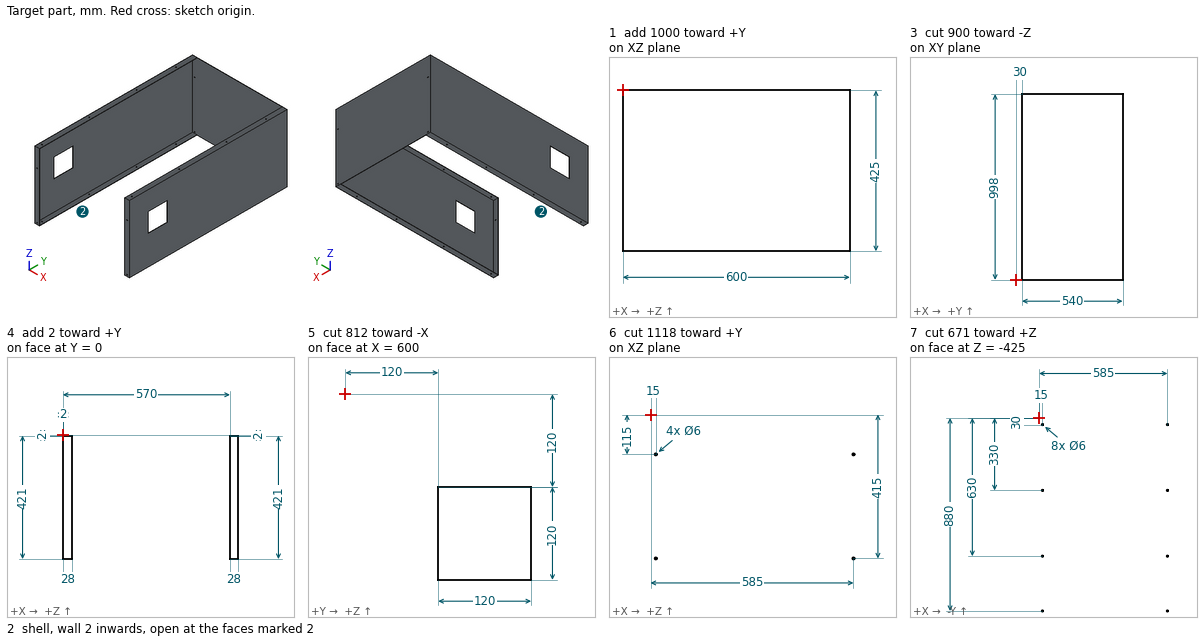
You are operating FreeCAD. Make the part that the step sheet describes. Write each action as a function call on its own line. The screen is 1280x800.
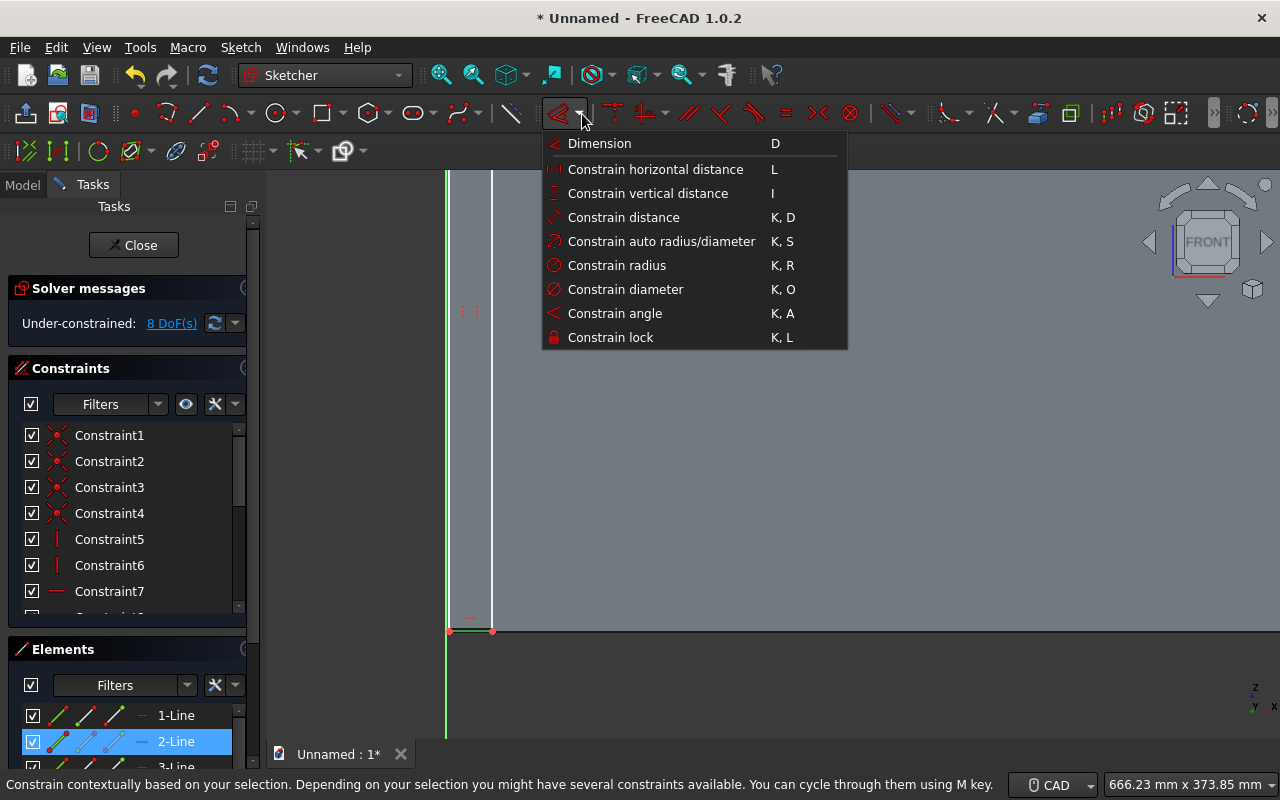
click(695, 169)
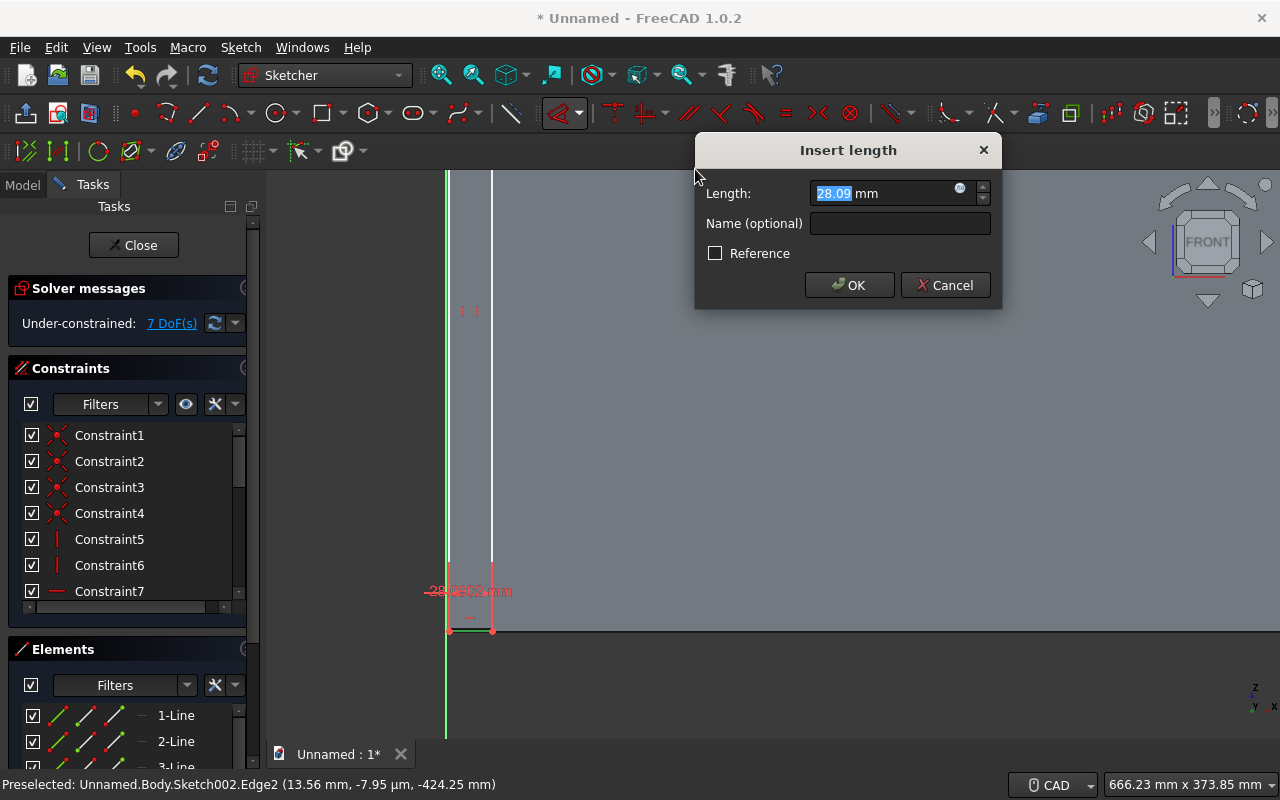
text(28)
key(Return)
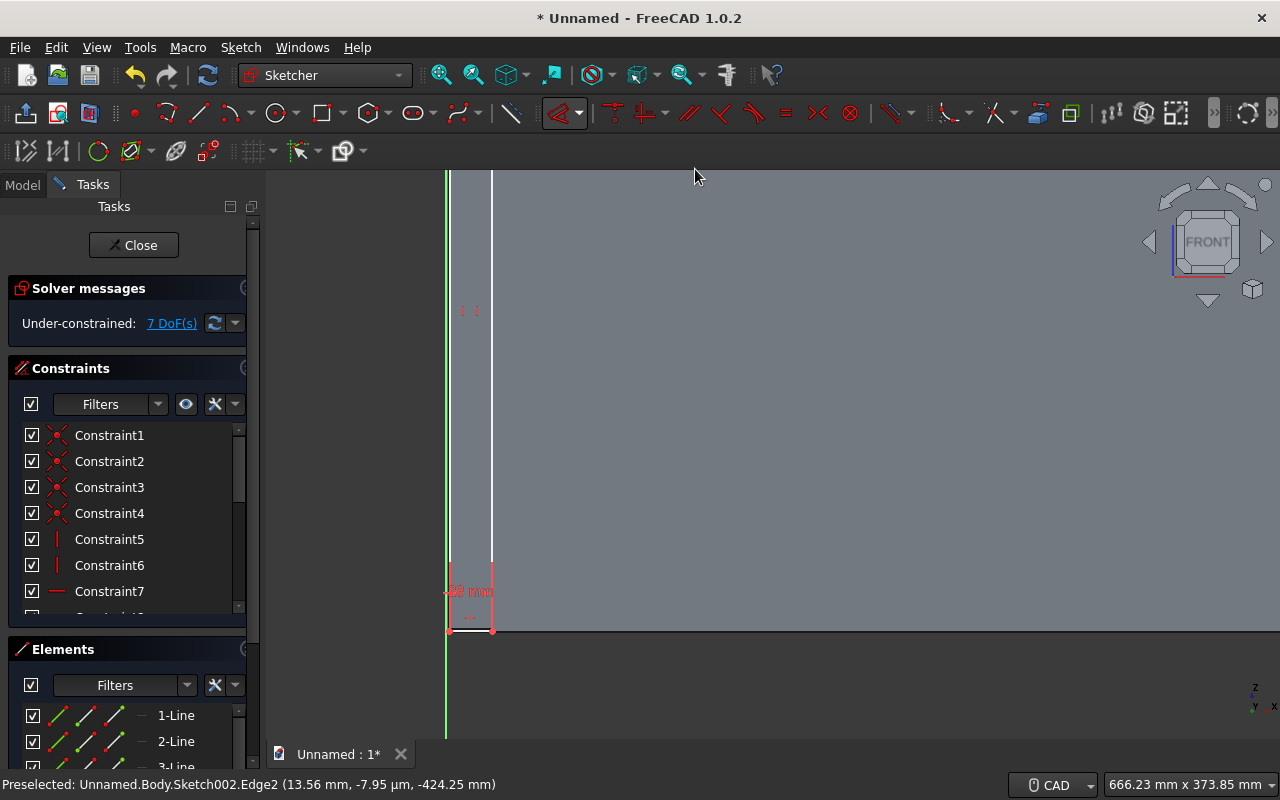
scroll(465, 633, down, 3)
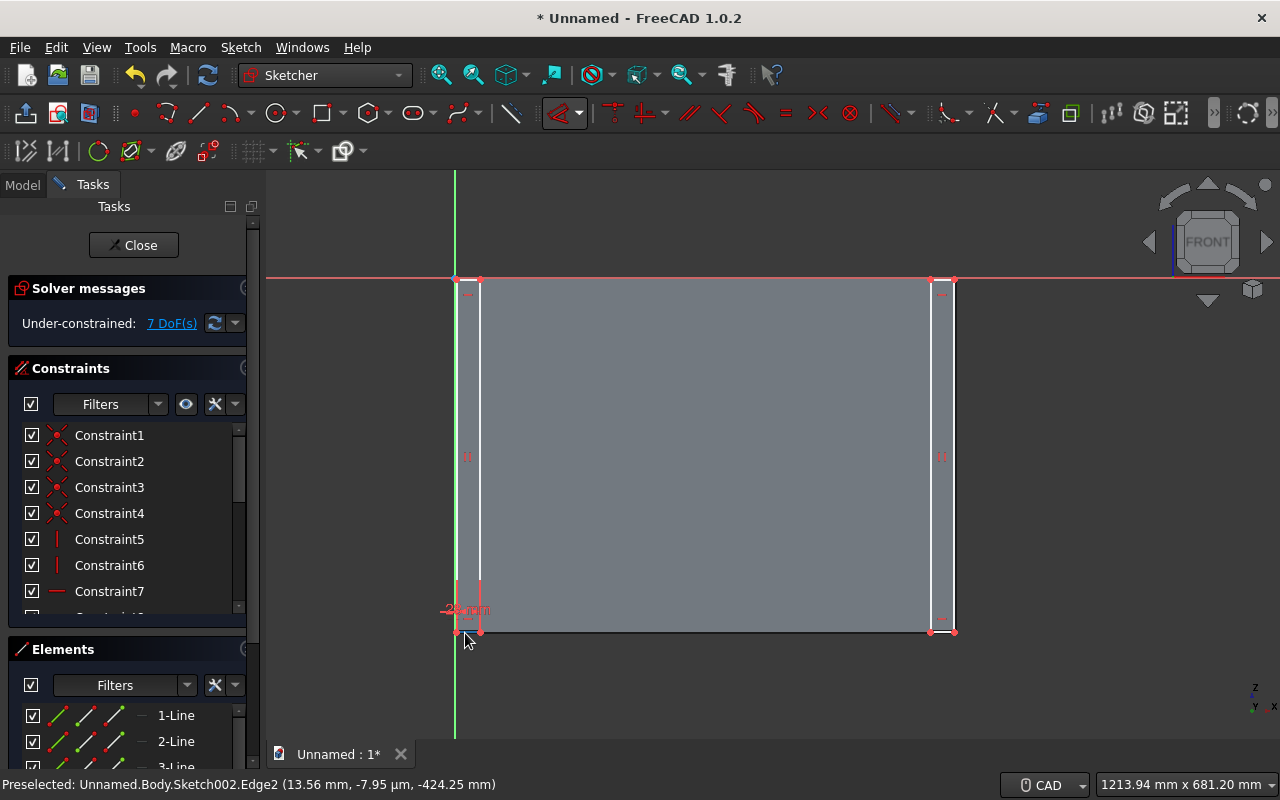
scroll(938, 632, up, 4)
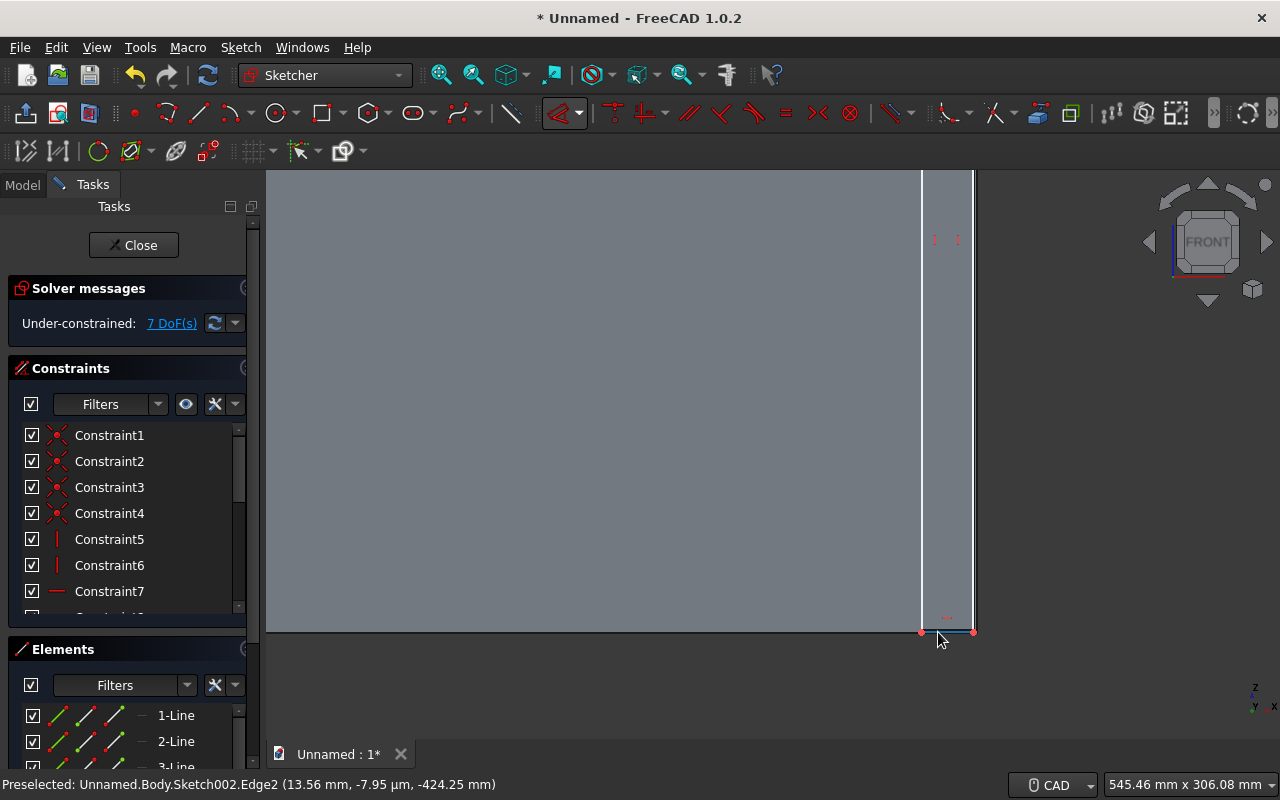
click(937, 632)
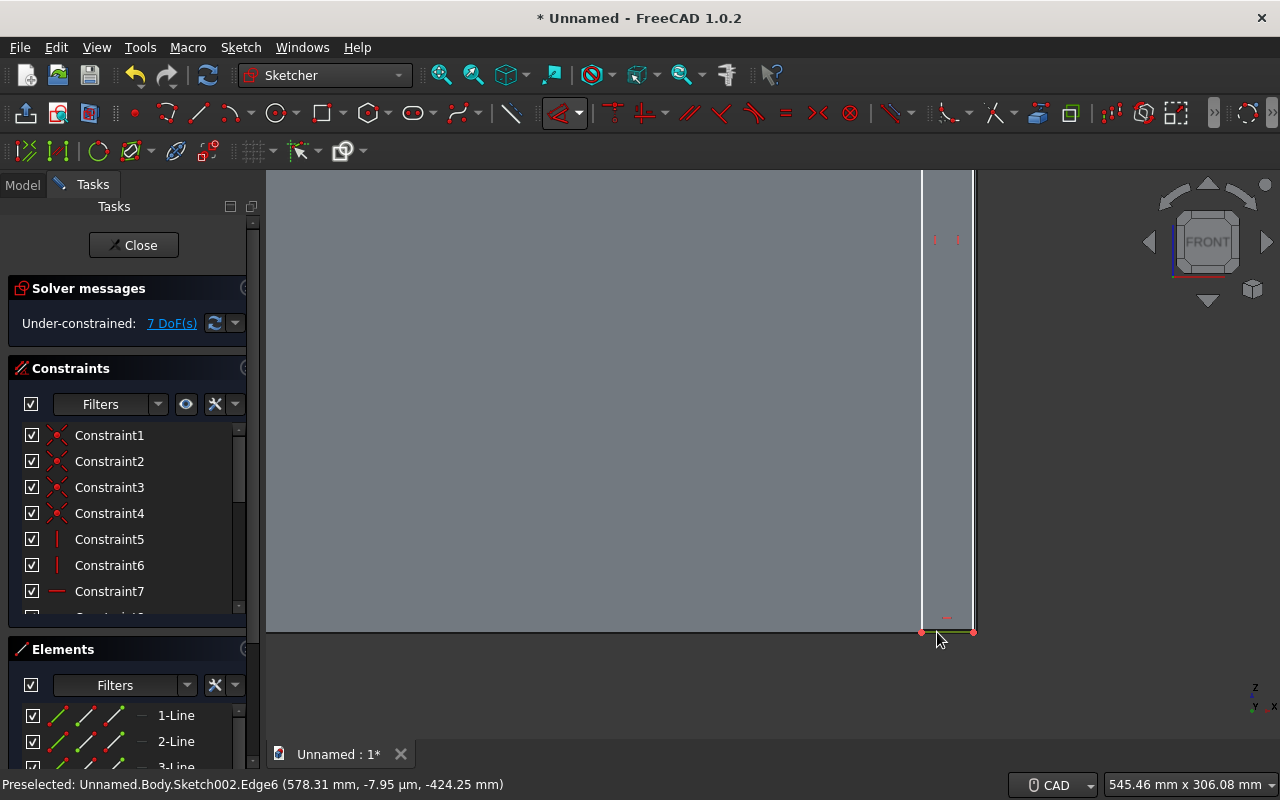
key(l)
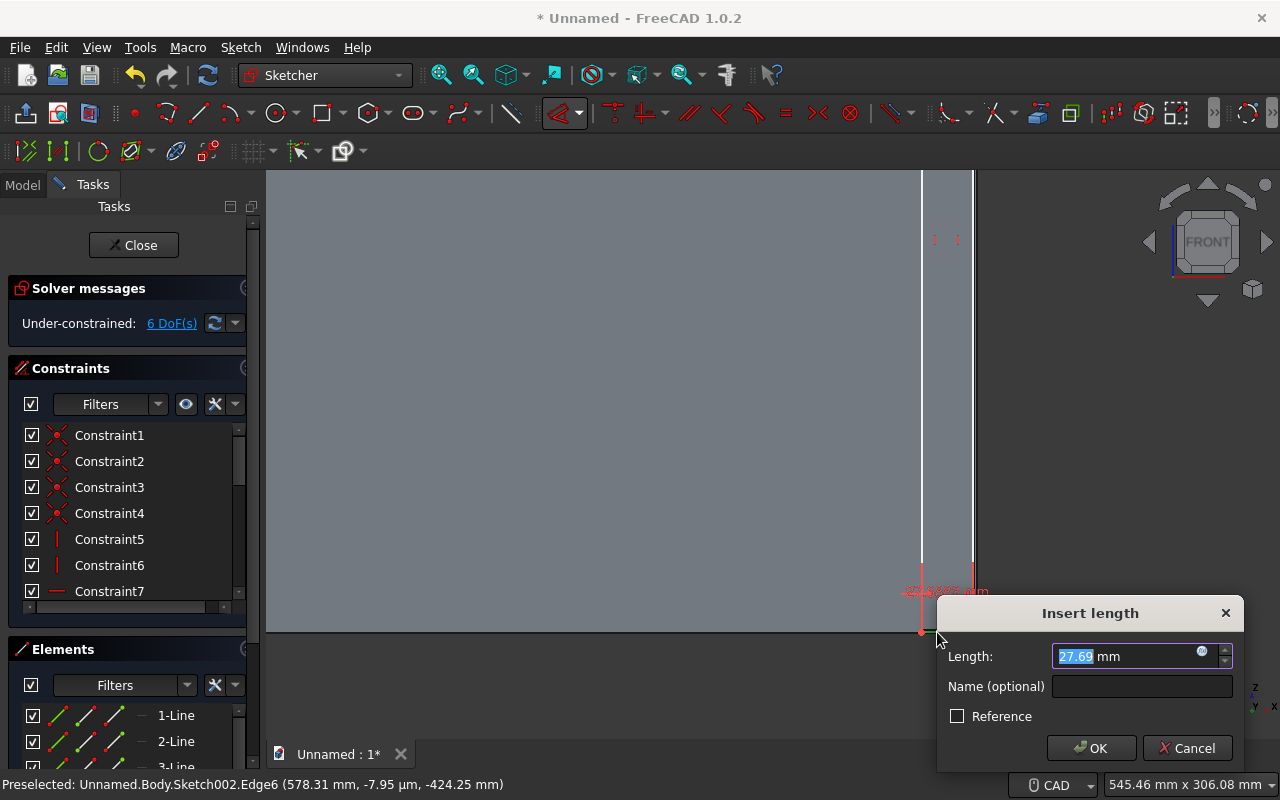
text(28)
key(Return)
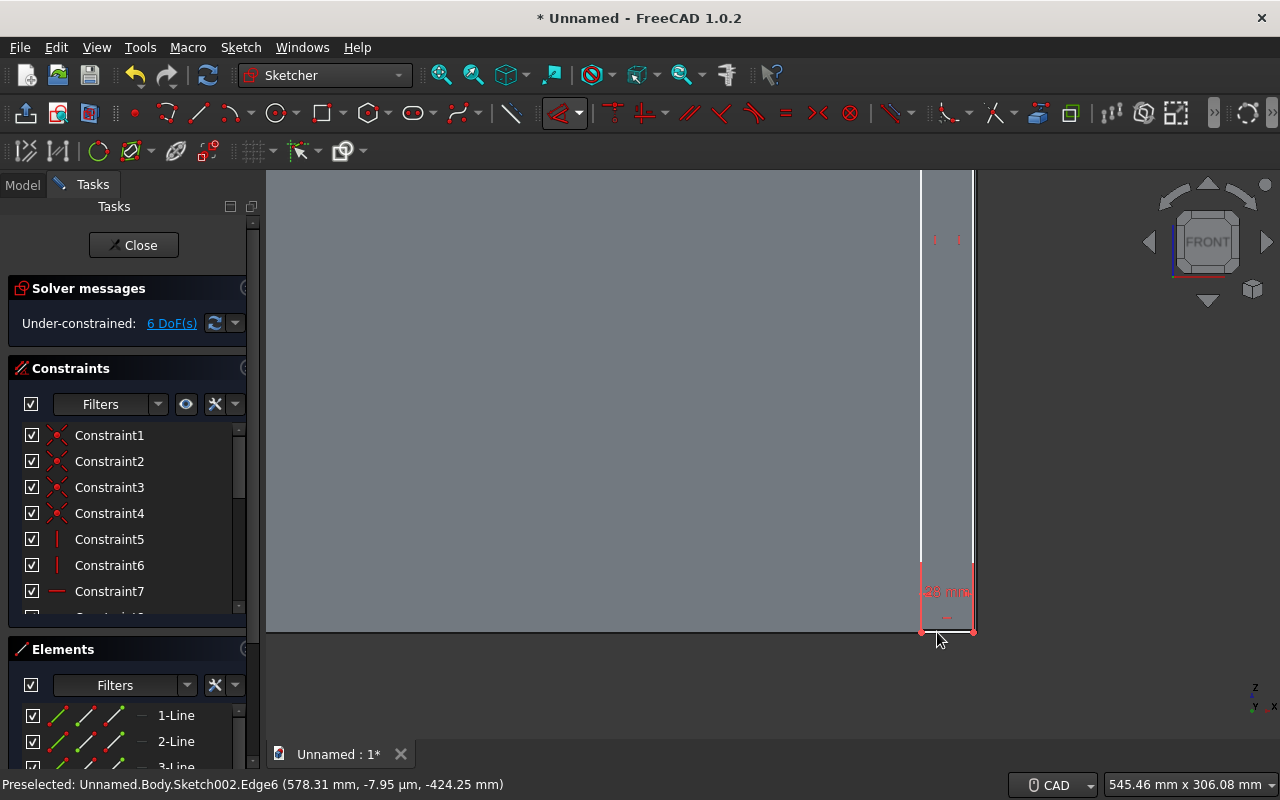
scroll(938, 632, down, 4)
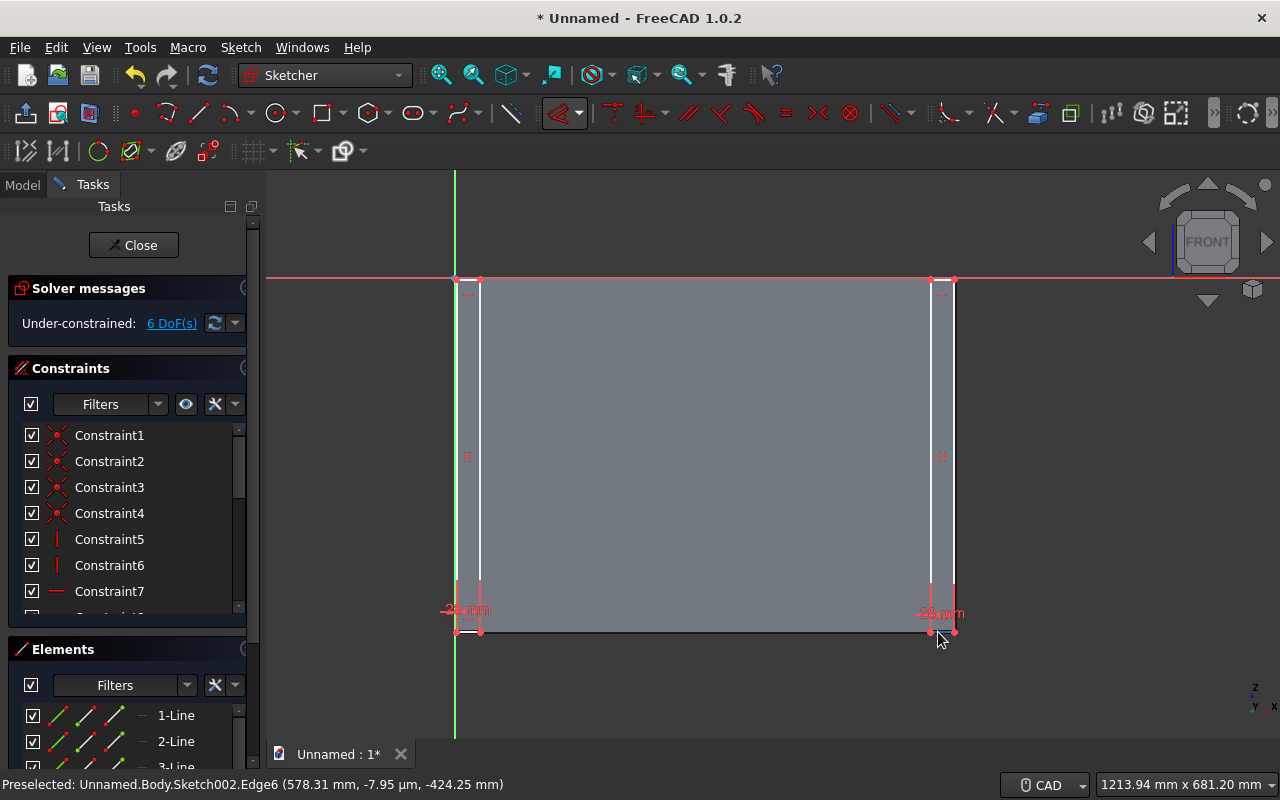
scroll(457, 280, up, 16)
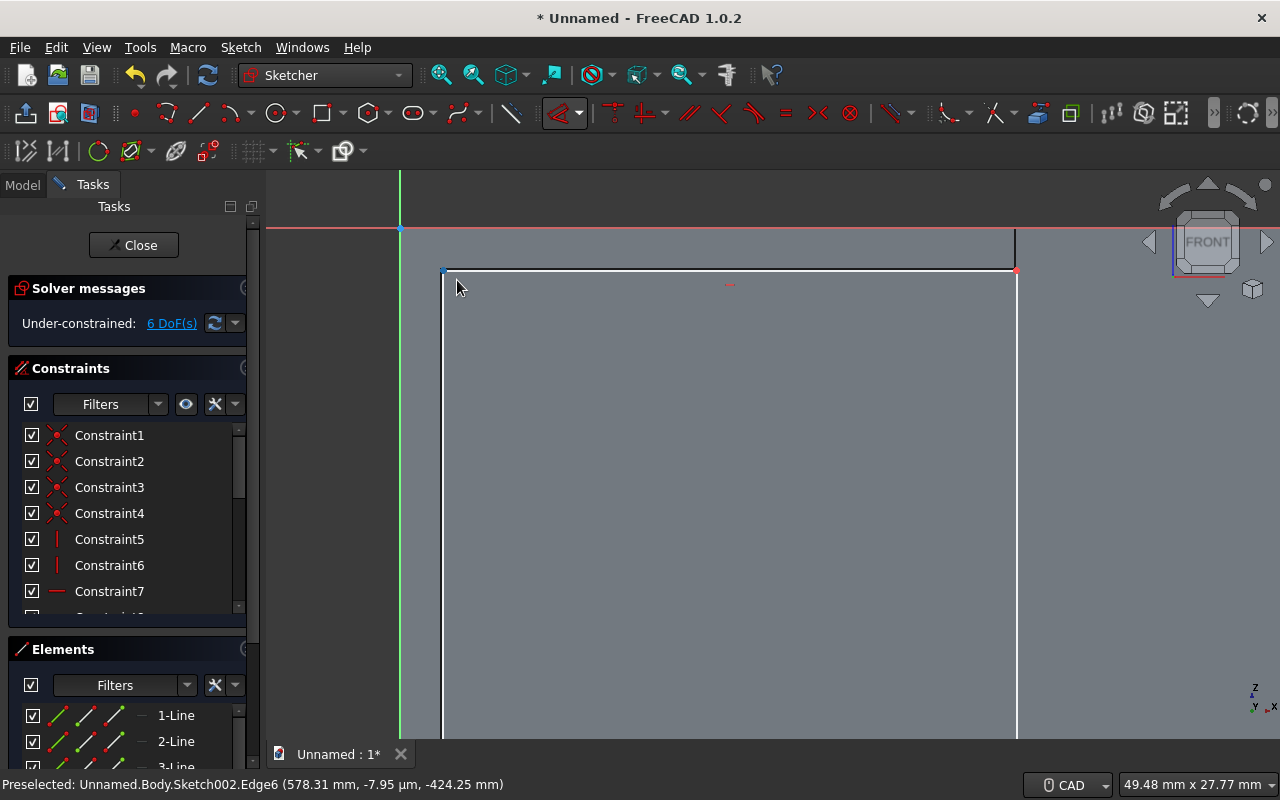
click(443, 271)